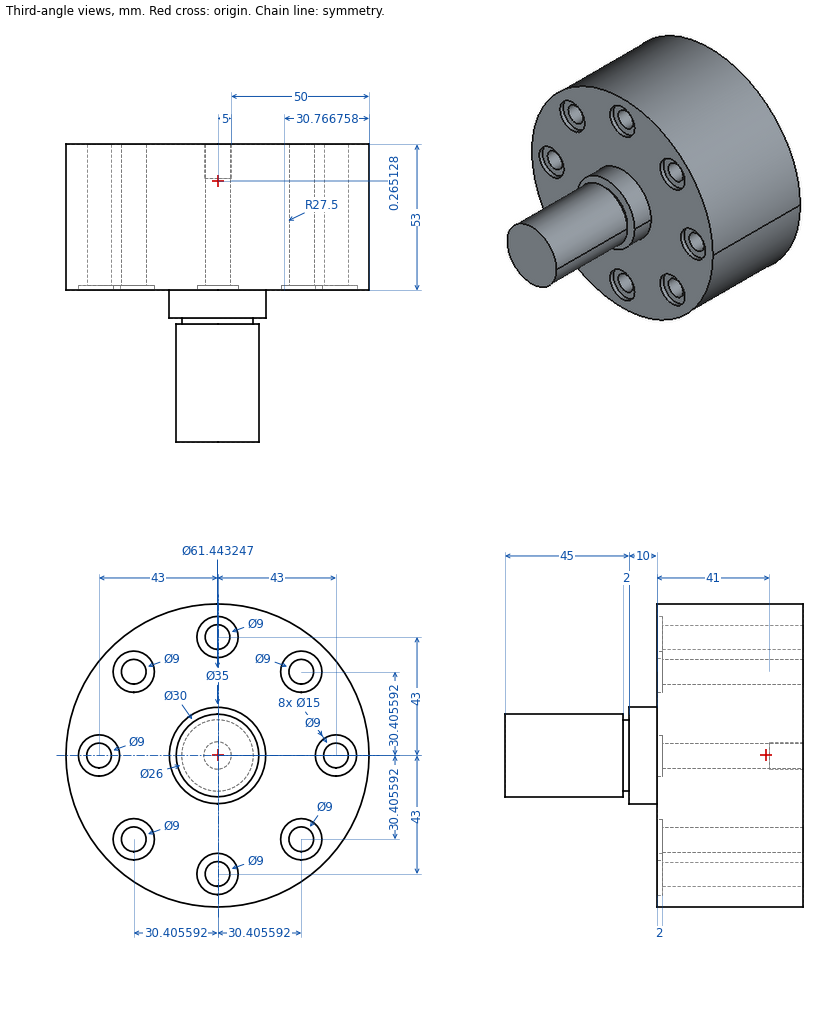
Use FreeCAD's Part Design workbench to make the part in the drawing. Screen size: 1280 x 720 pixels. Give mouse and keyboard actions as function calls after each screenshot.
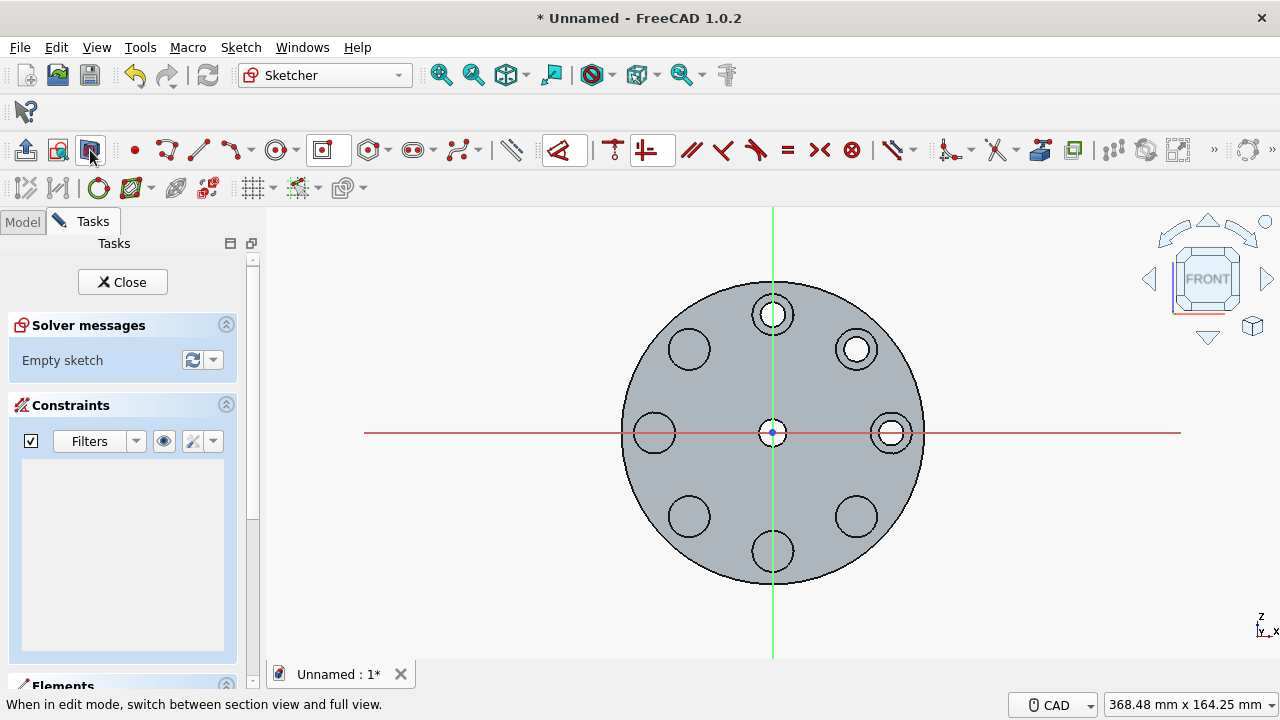
scroll(872, 525, up, 12)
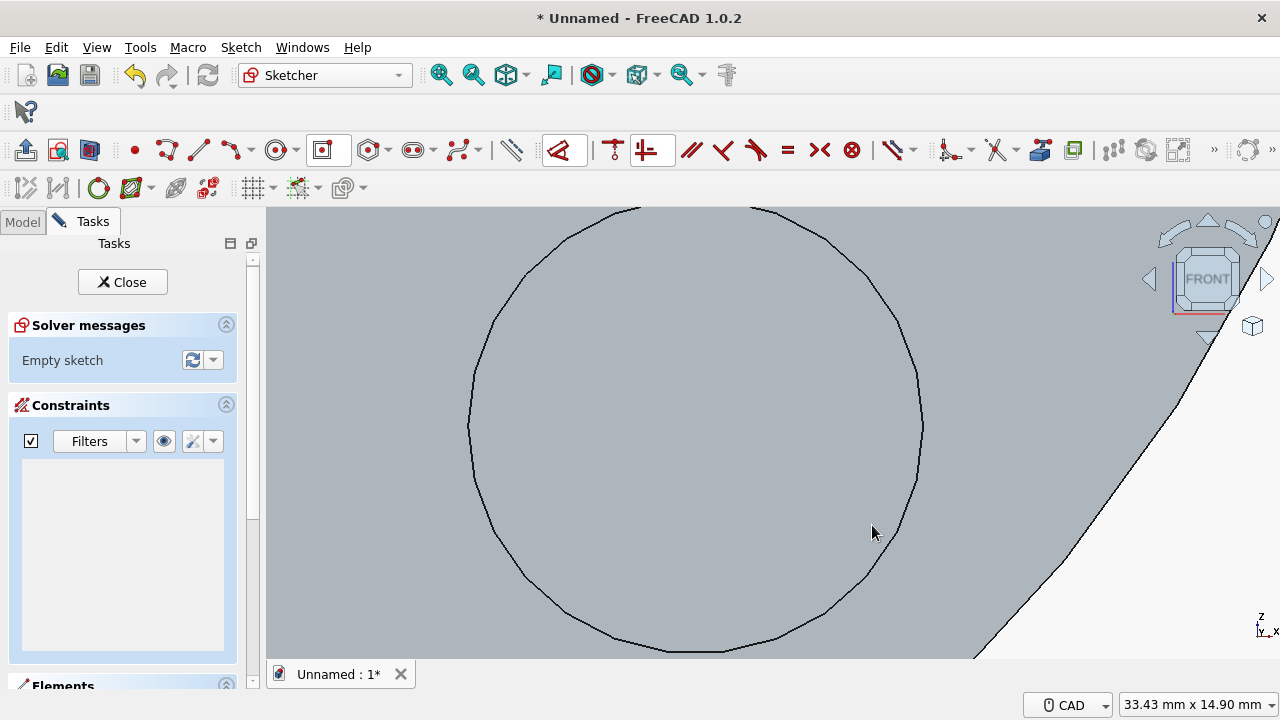
click(276, 150)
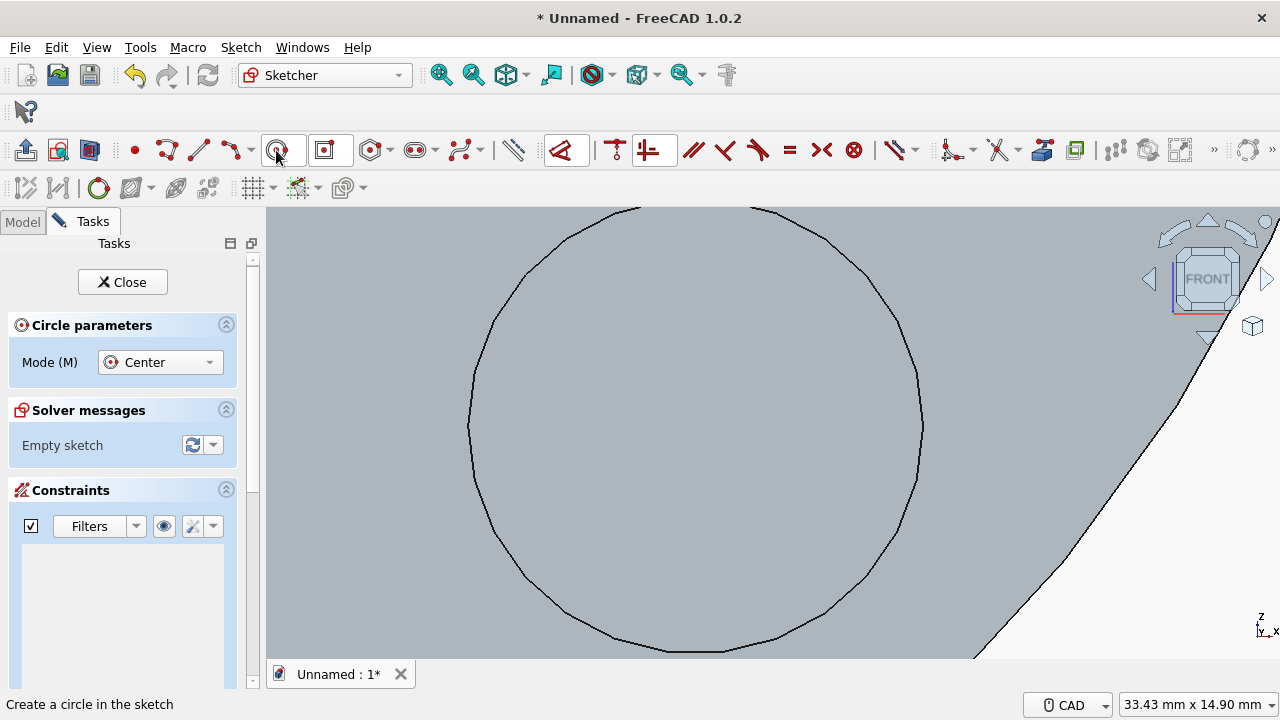
click(696, 426)
move(792, 330)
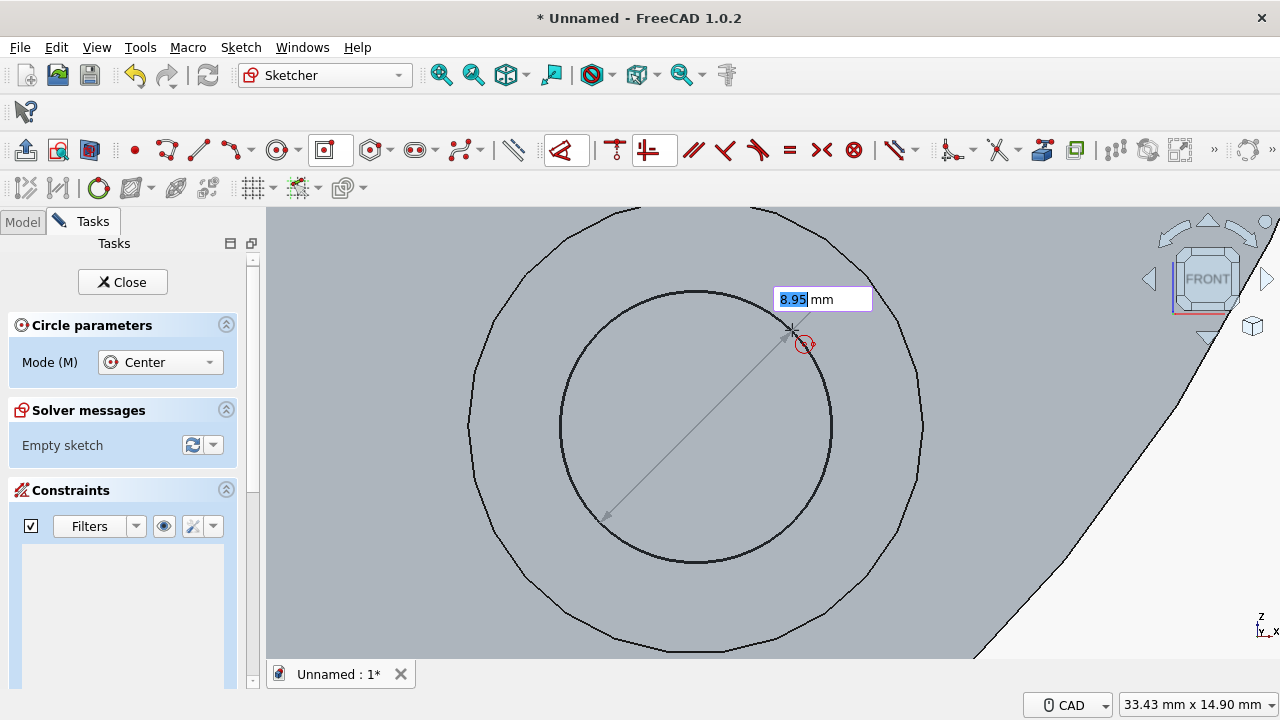
text(9)
key(Return)
key(Escape)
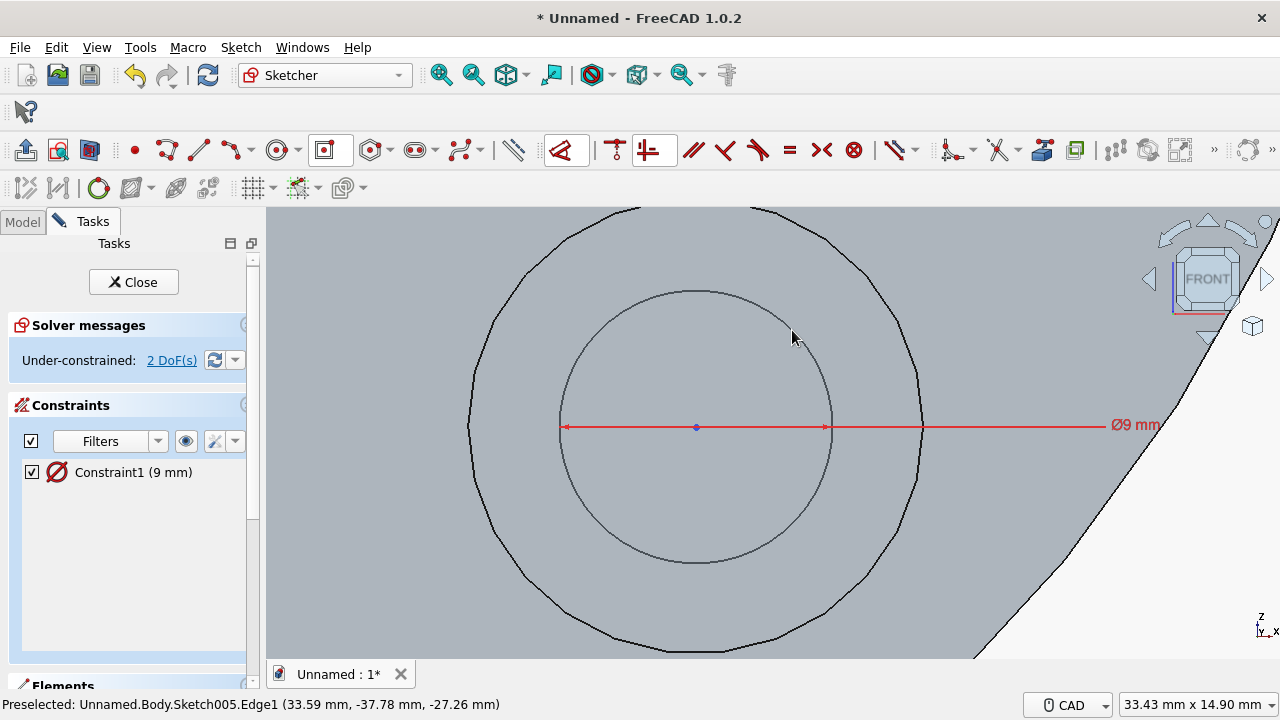
click(696, 427)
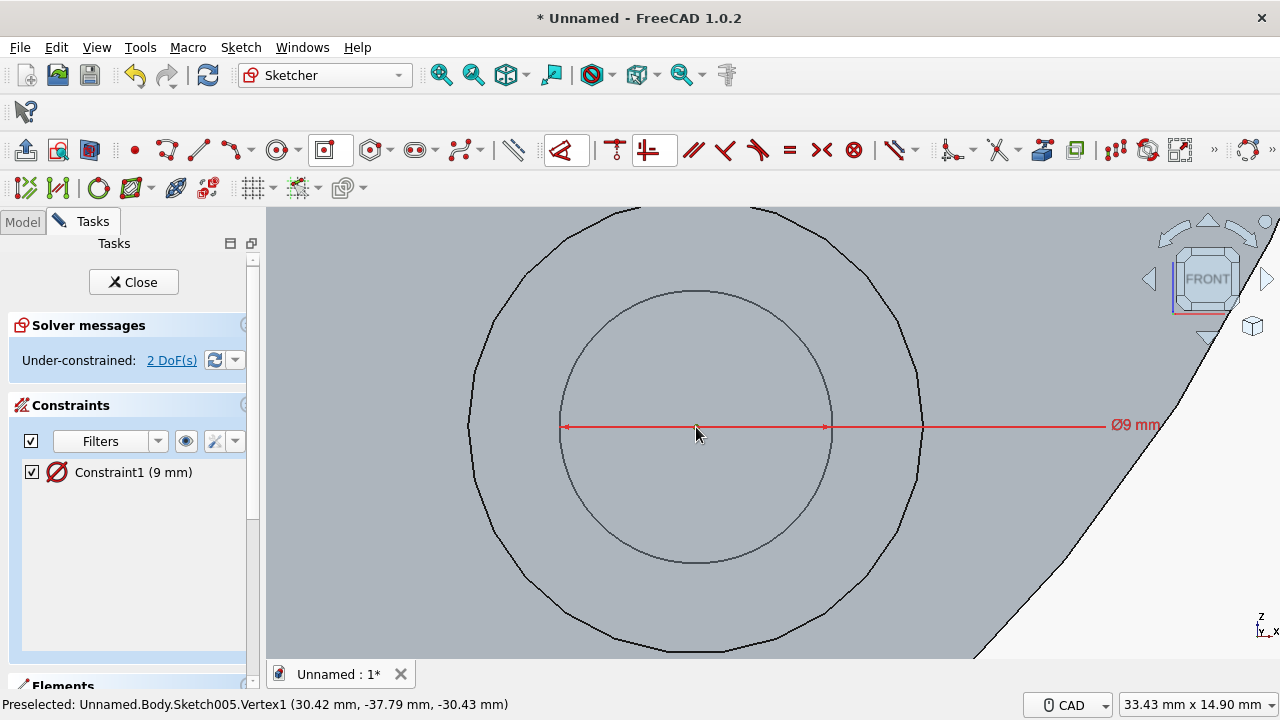
click(584, 150)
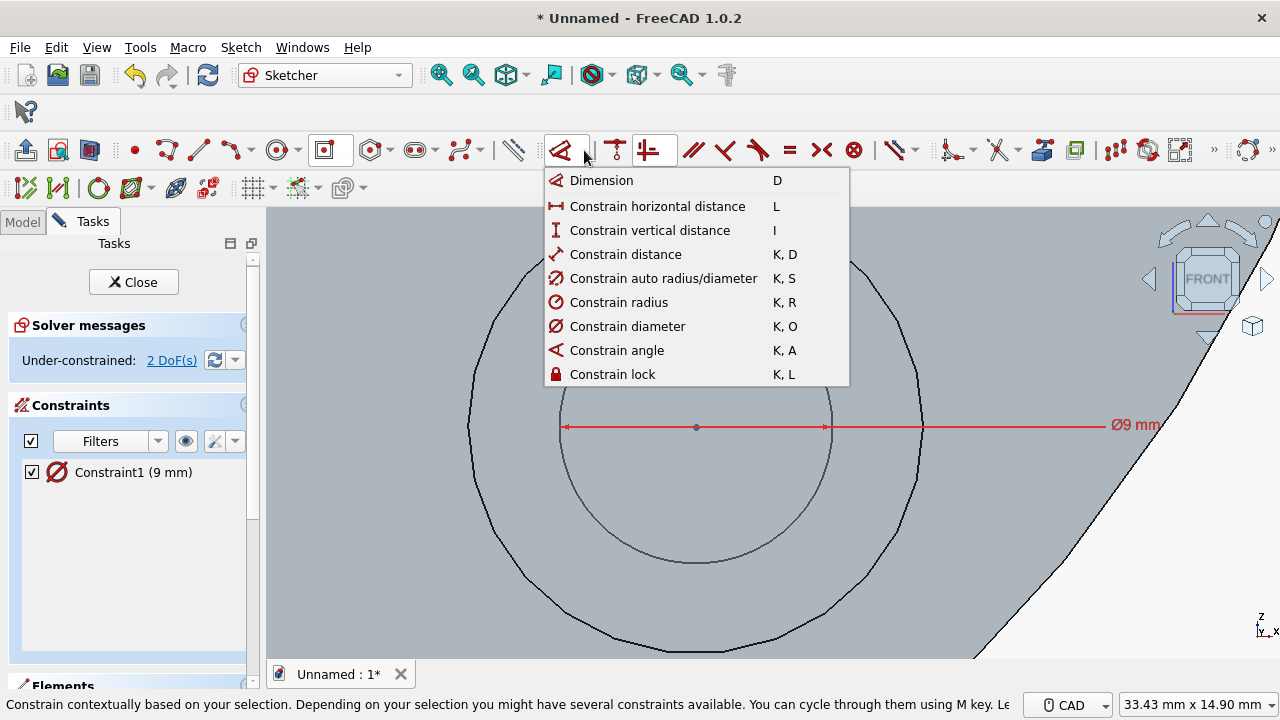
click(697, 206)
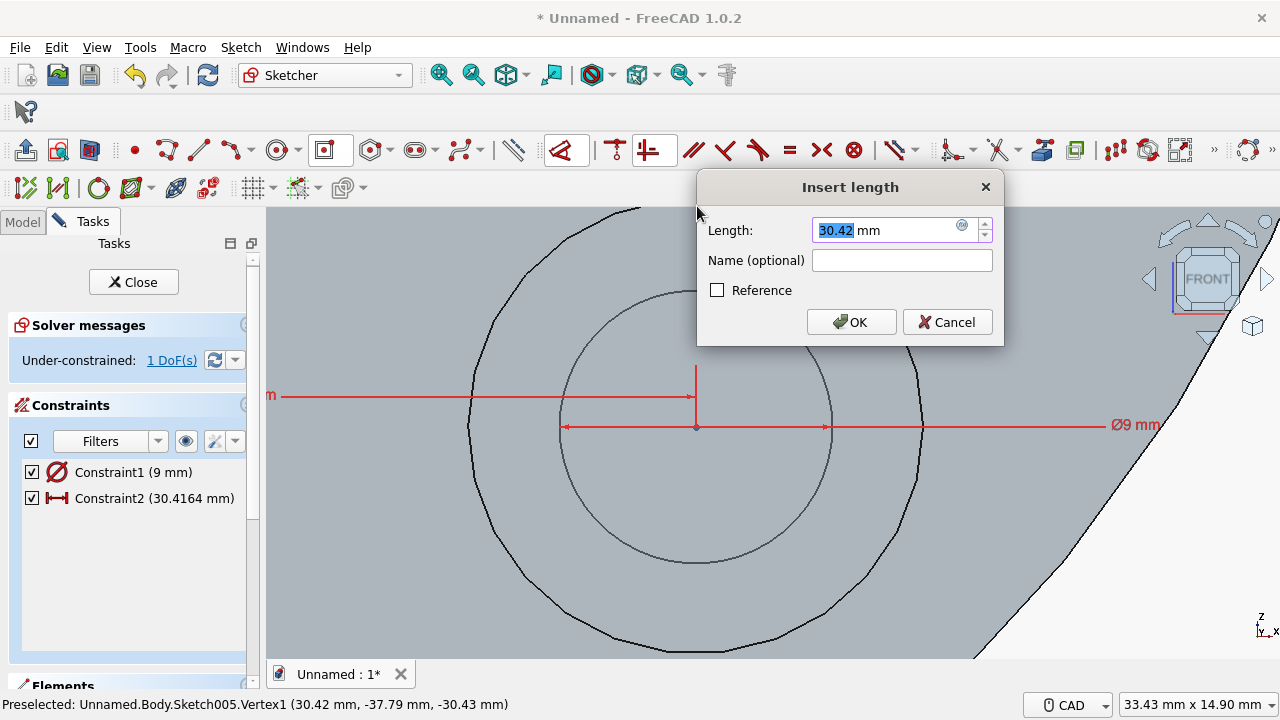
text(30.405592)
key(Return)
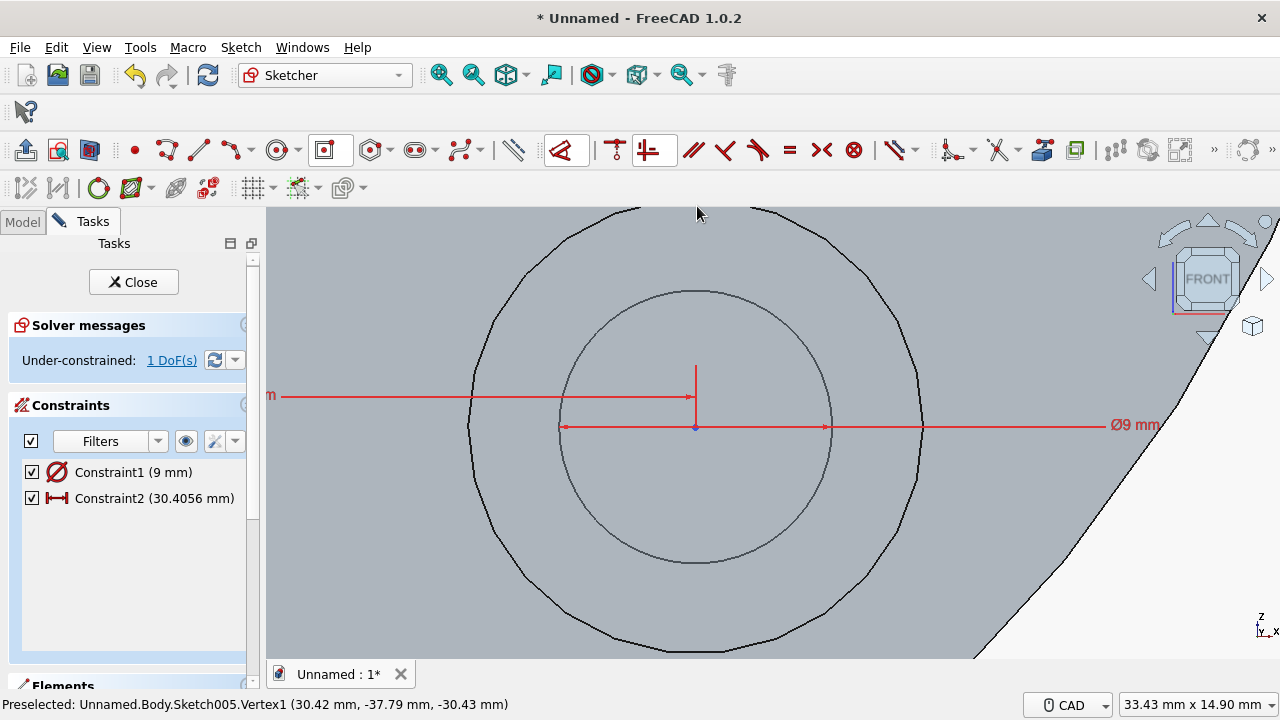
click(696, 427)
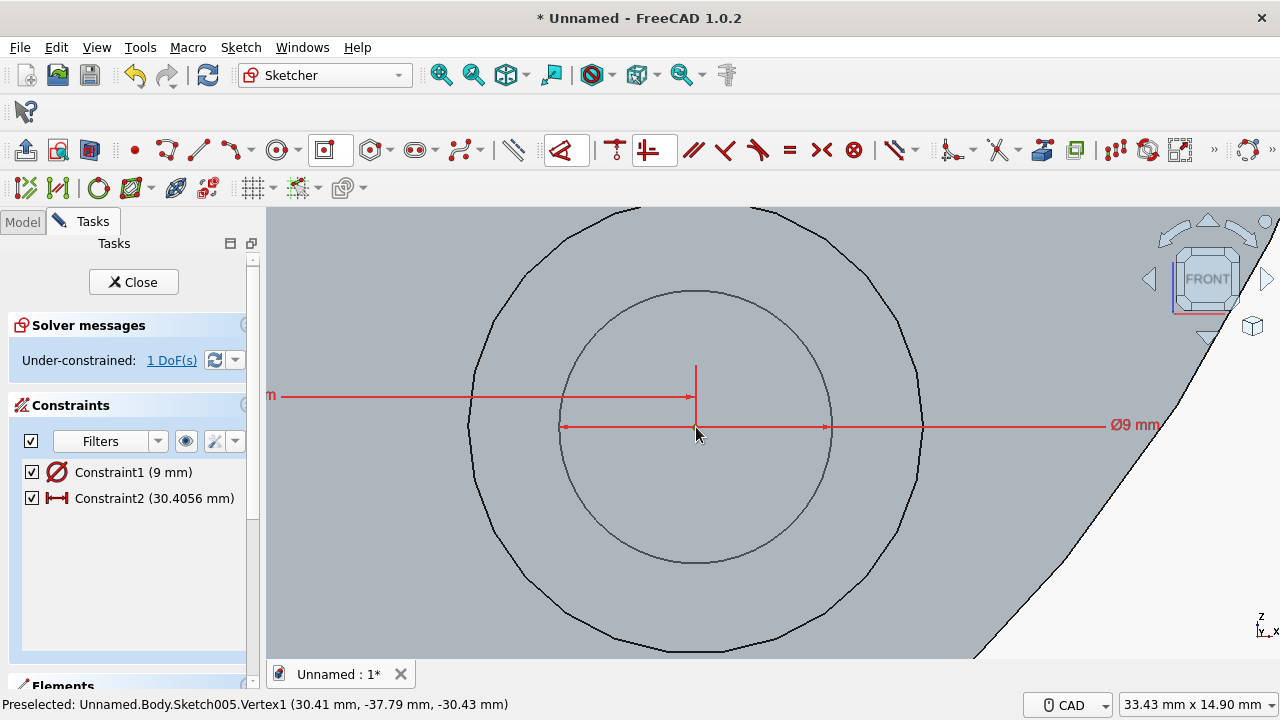
click(584, 150)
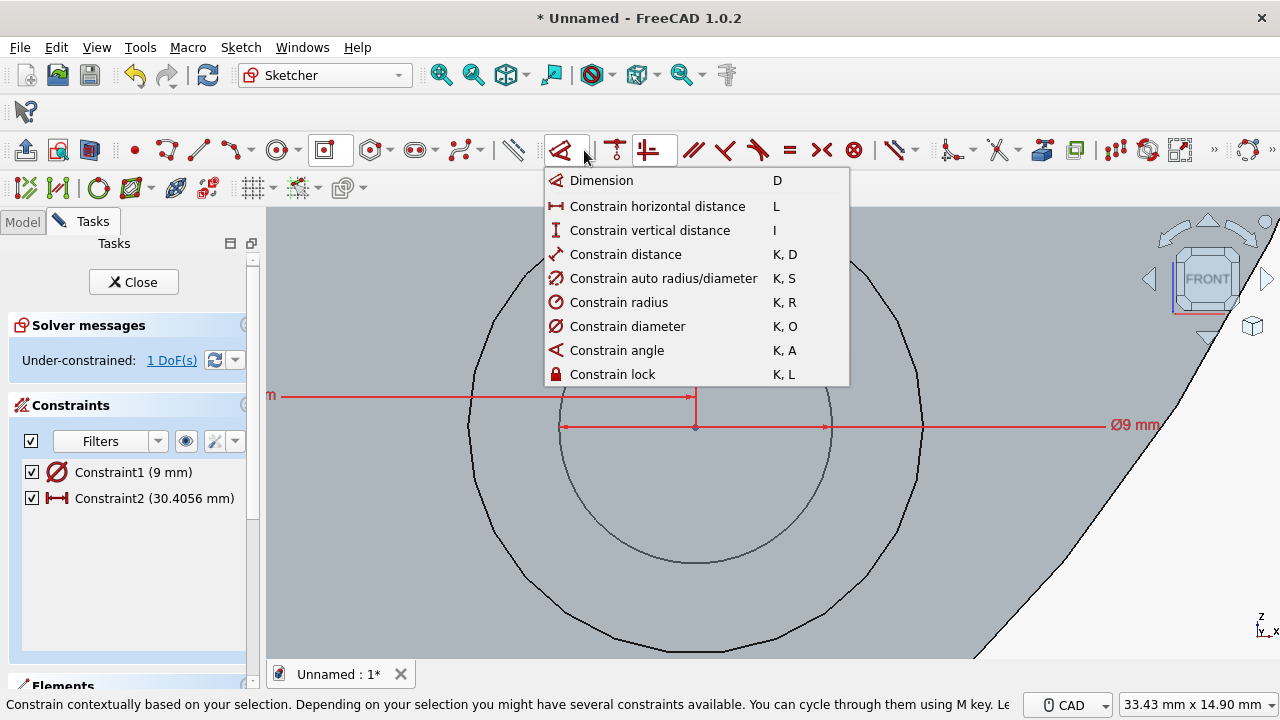
click(697, 230)